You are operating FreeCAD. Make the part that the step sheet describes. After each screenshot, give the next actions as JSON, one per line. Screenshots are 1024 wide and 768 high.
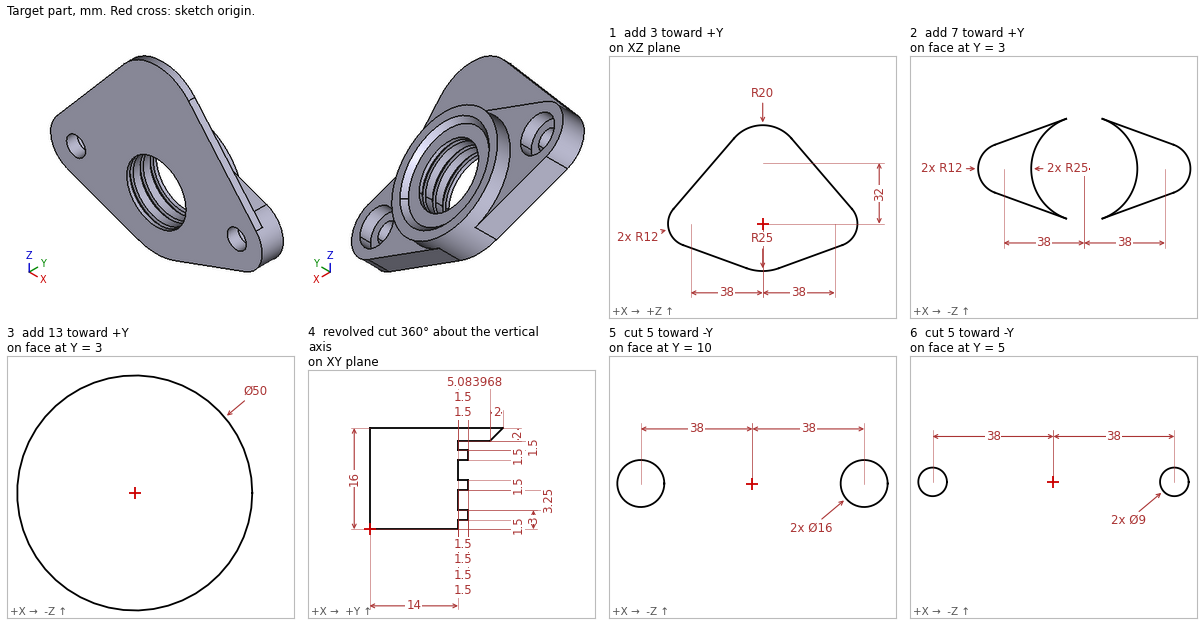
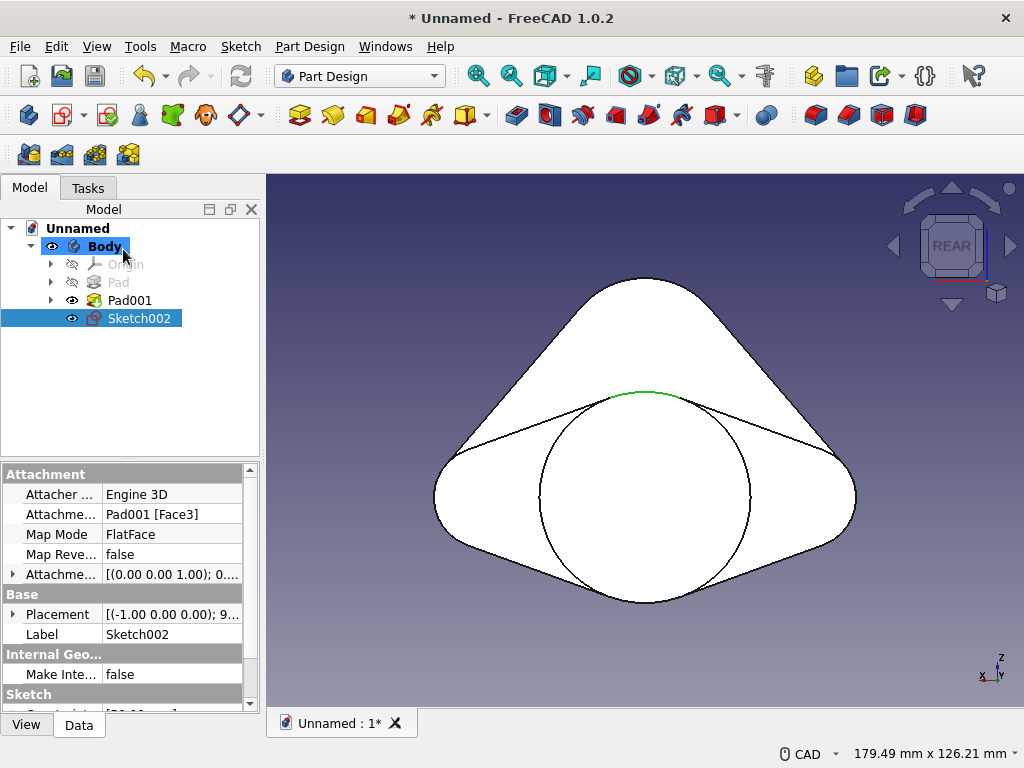
{"action": "left_click", "coordinate": [300, 116]}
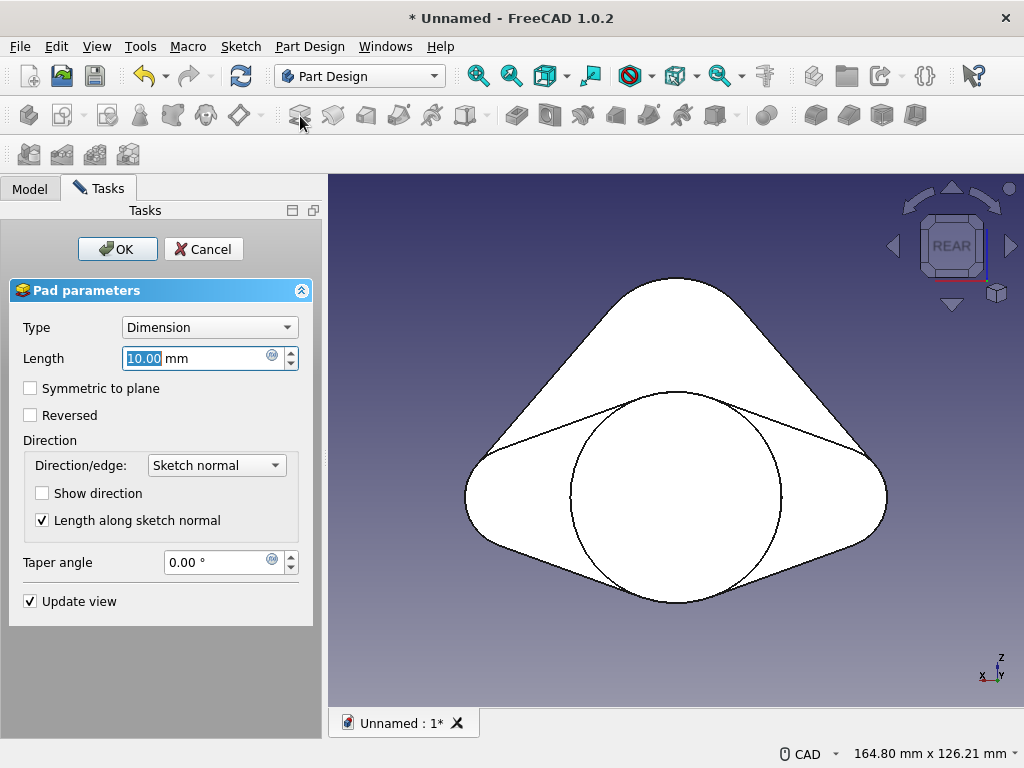
{"action": "type", "text": "13"}
{"action": "key", "text": "Tab"}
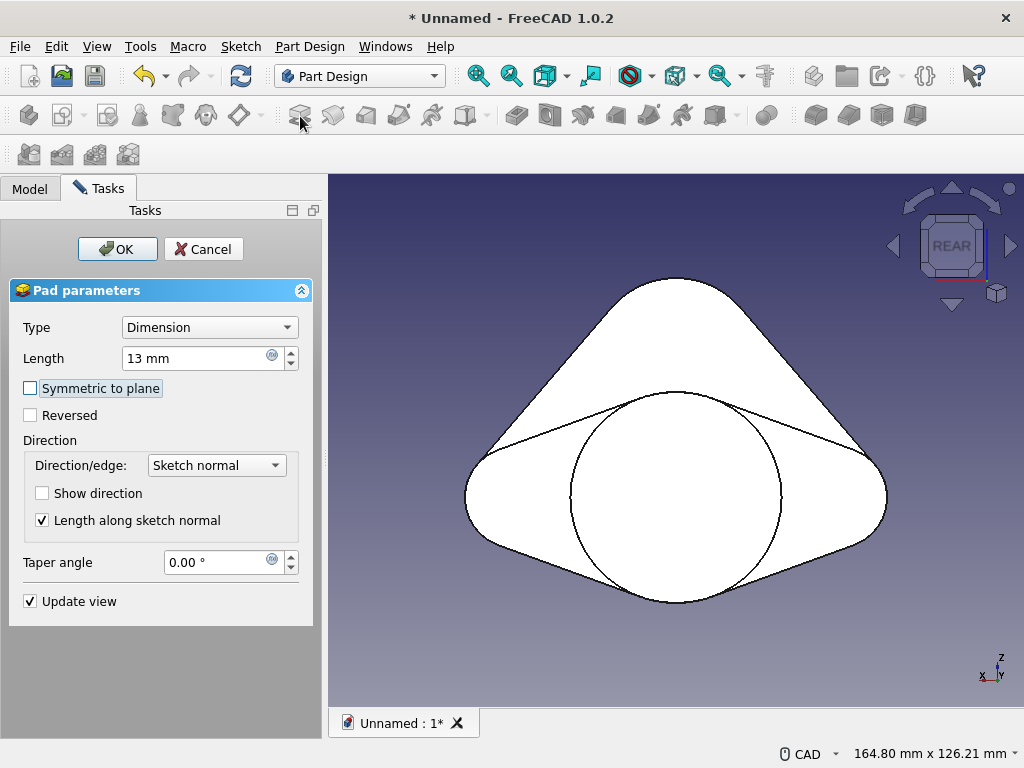
{"action": "left_click", "coordinate": [118, 249]}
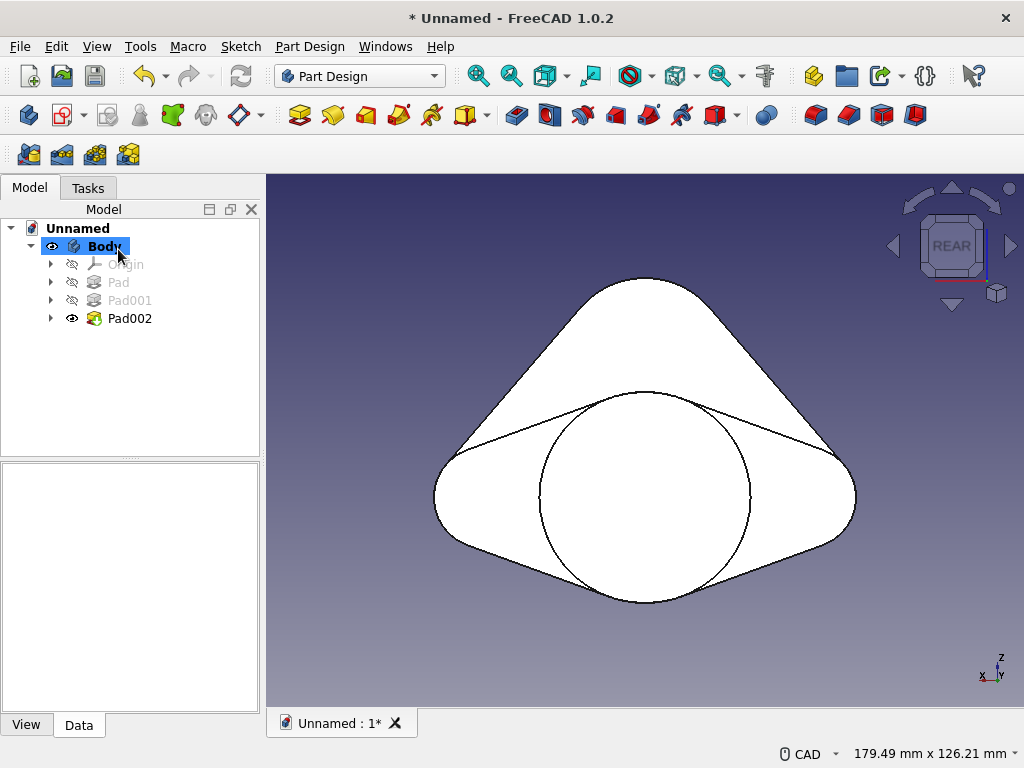
{"action": "left_click", "coordinate": [62, 116]}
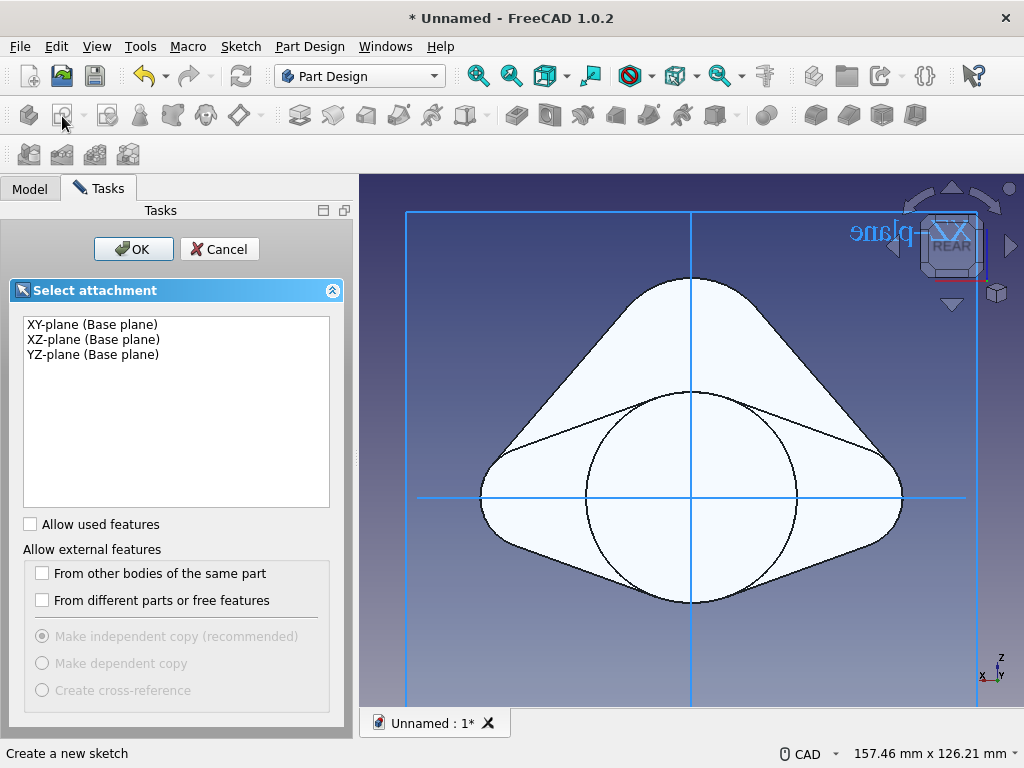
{"action": "left_click", "coordinate": [84, 324]}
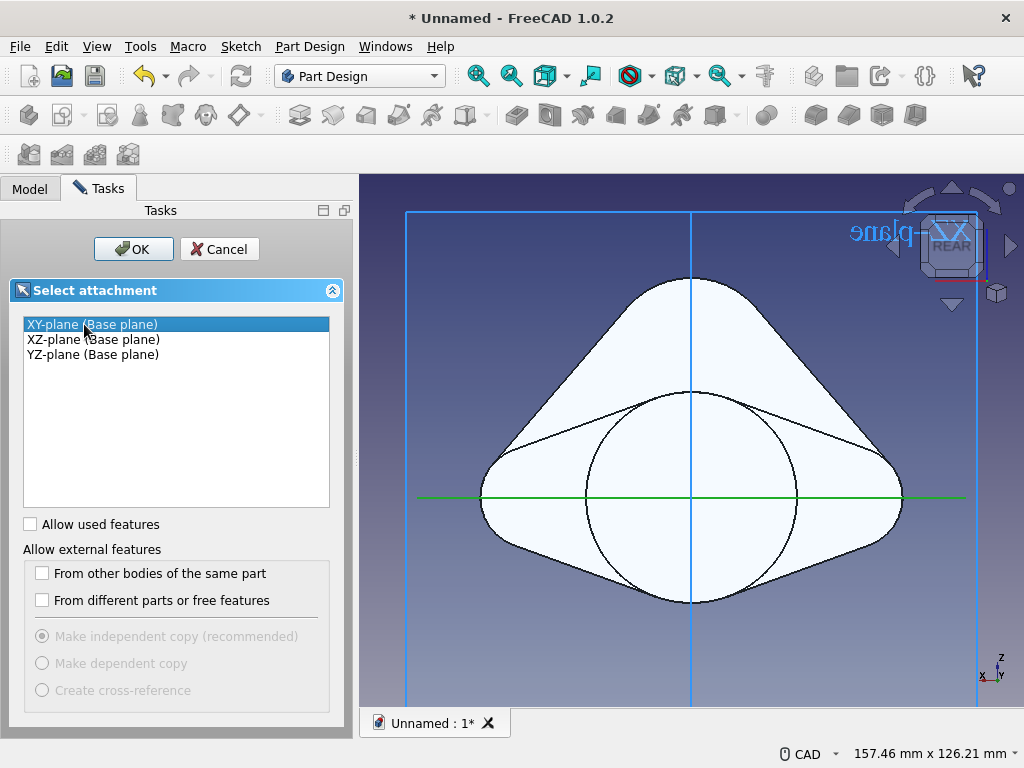
{"action": "left_click", "coordinate": [134, 249]}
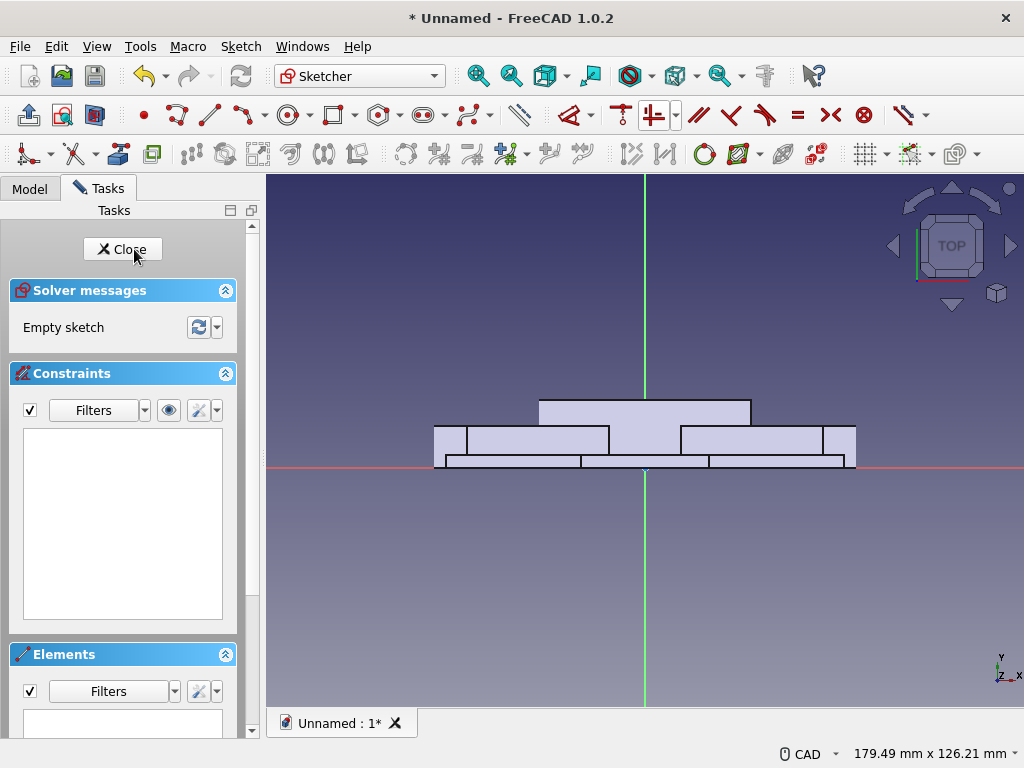
{"action": "left_click", "coordinate": [95, 116]}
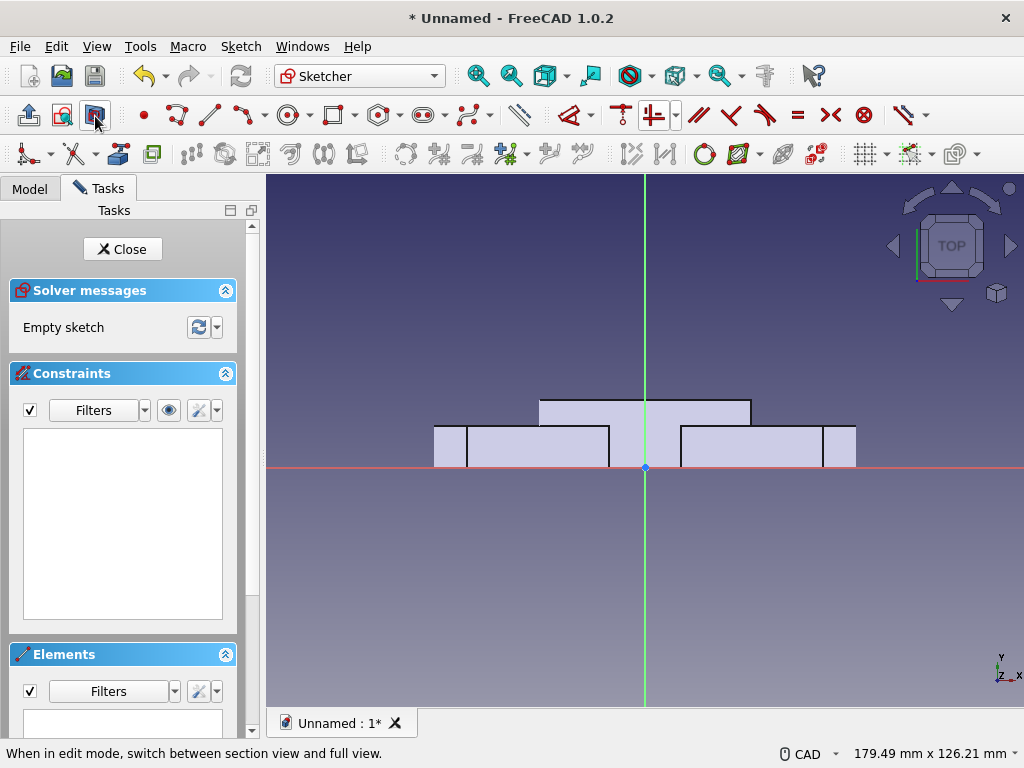
{"action": "scroll", "coordinate": [727, 432], "scroll_direction": "up", "scroll_amount": 7}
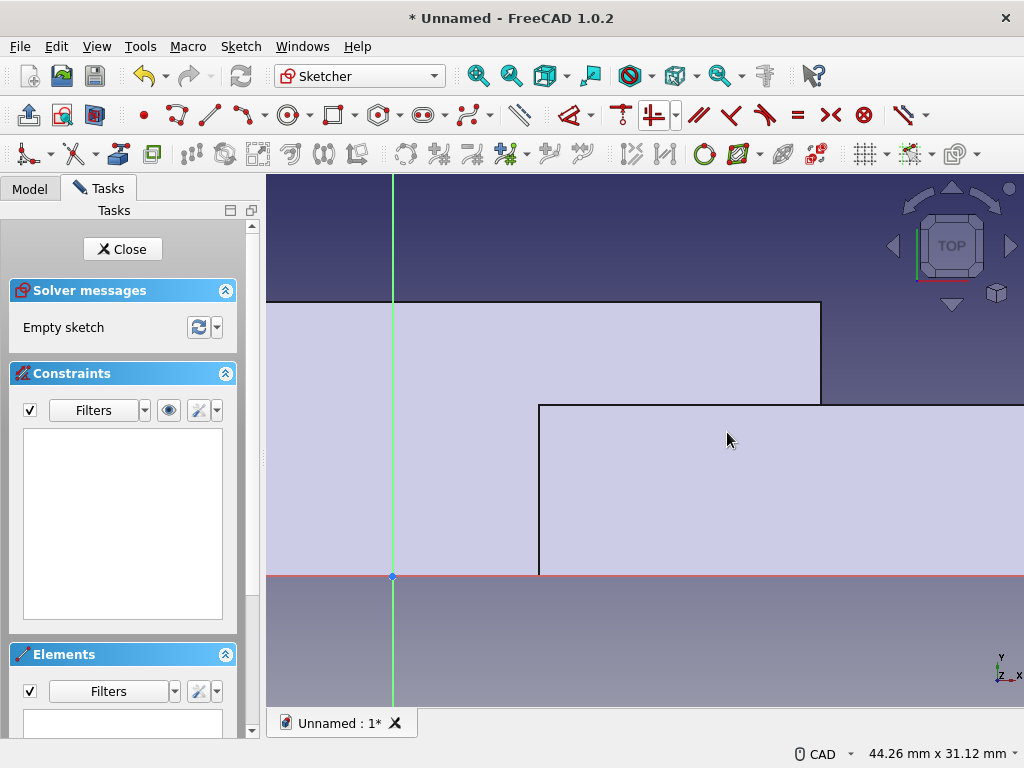
{"action": "left_click", "coordinate": [177, 116]}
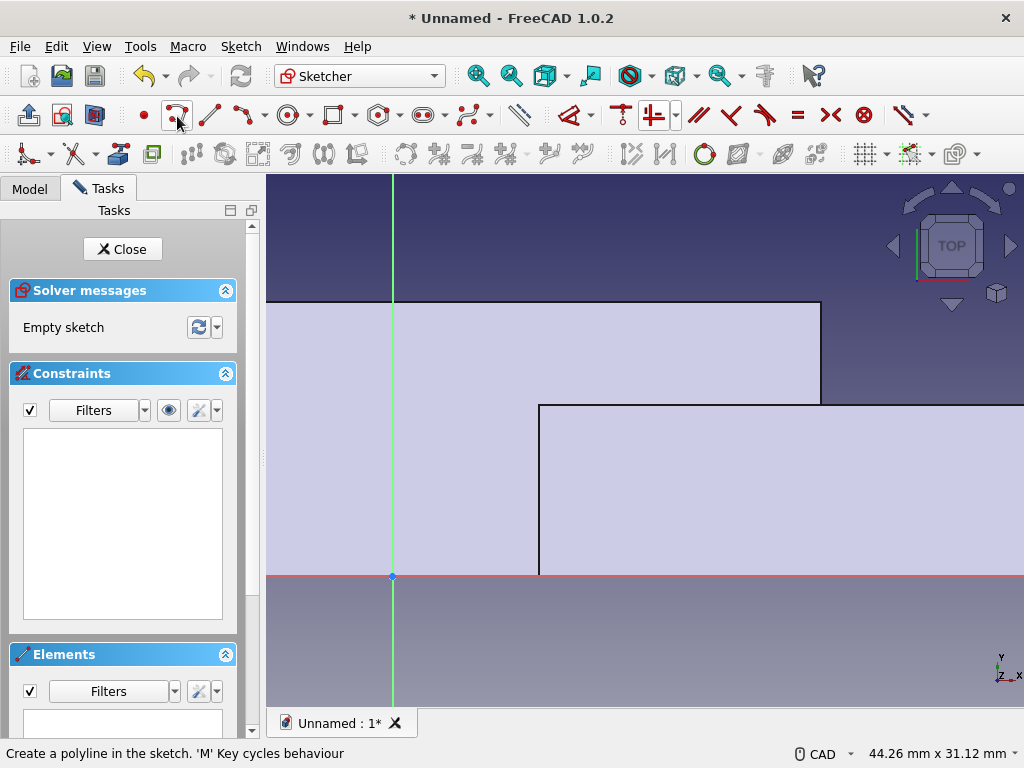
{"action": "left_click", "coordinate": [393, 576]}
{"action": "left_click", "coordinate": [632, 567]}
{"action": "left_click", "coordinate": [632, 551]}
{"action": "left_click", "coordinate": [658, 551]}
{"action": "left_click", "coordinate": [658, 525]}
{"action": "left_click", "coordinate": [632, 525]}
{"action": "left_click", "coordinate": [632, 469]}
{"action": "left_click", "coordinate": [658, 469]}
{"action": "left_click", "coordinate": [658, 444]}
{"action": "left_click", "coordinate": [632, 444]}
{"action": "left_click", "coordinate": [632, 388]}
{"action": "left_click", "coordinate": [658, 388]}
{"action": "left_click", "coordinate": [658, 362]}
{"action": "left_click", "coordinate": [632, 362]}
{"action": "left_click", "coordinate": [632, 337]}
{"action": "left_click", "coordinate": [719, 337]}
{"action": "left_click", "coordinate": [754, 302]}
{"action": "left_click", "coordinate": [402, 302]}
{"action": "left_click", "coordinate": [393, 576]}
{"action": "key", "text": "Escape"}
{"action": "key", "text": "Escape"}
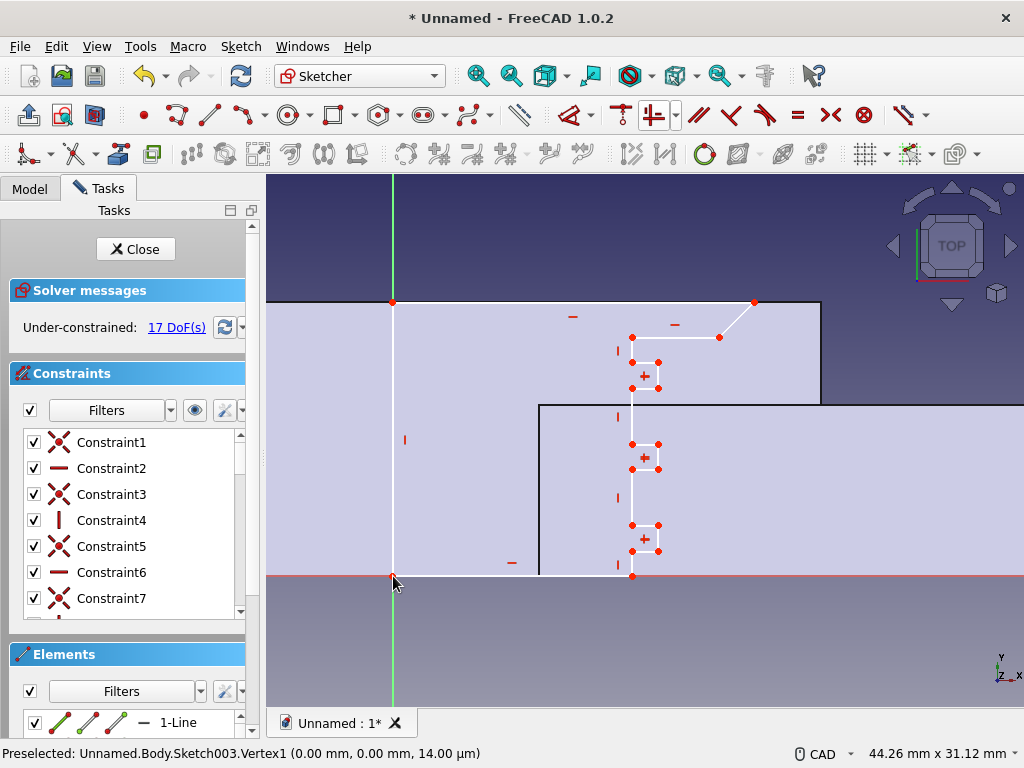
{"action": "left_click", "coordinate": [568, 116]}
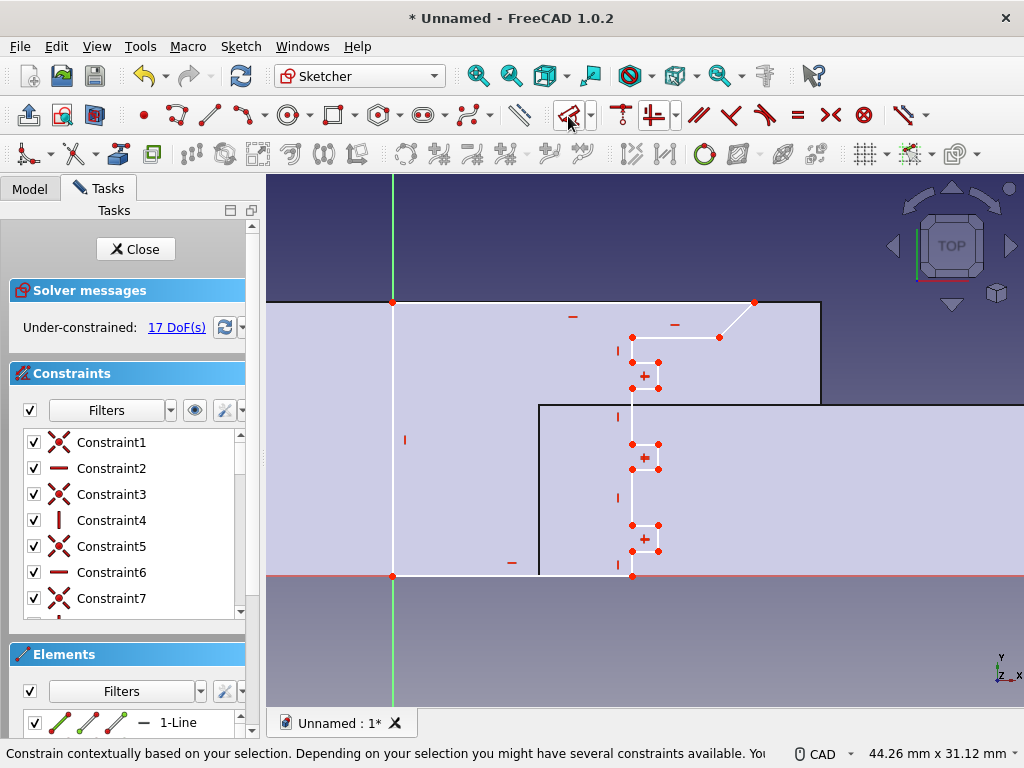
{"action": "left_click", "coordinate": [464, 576]}
{"action": "left_click", "coordinate": [512, 610]}